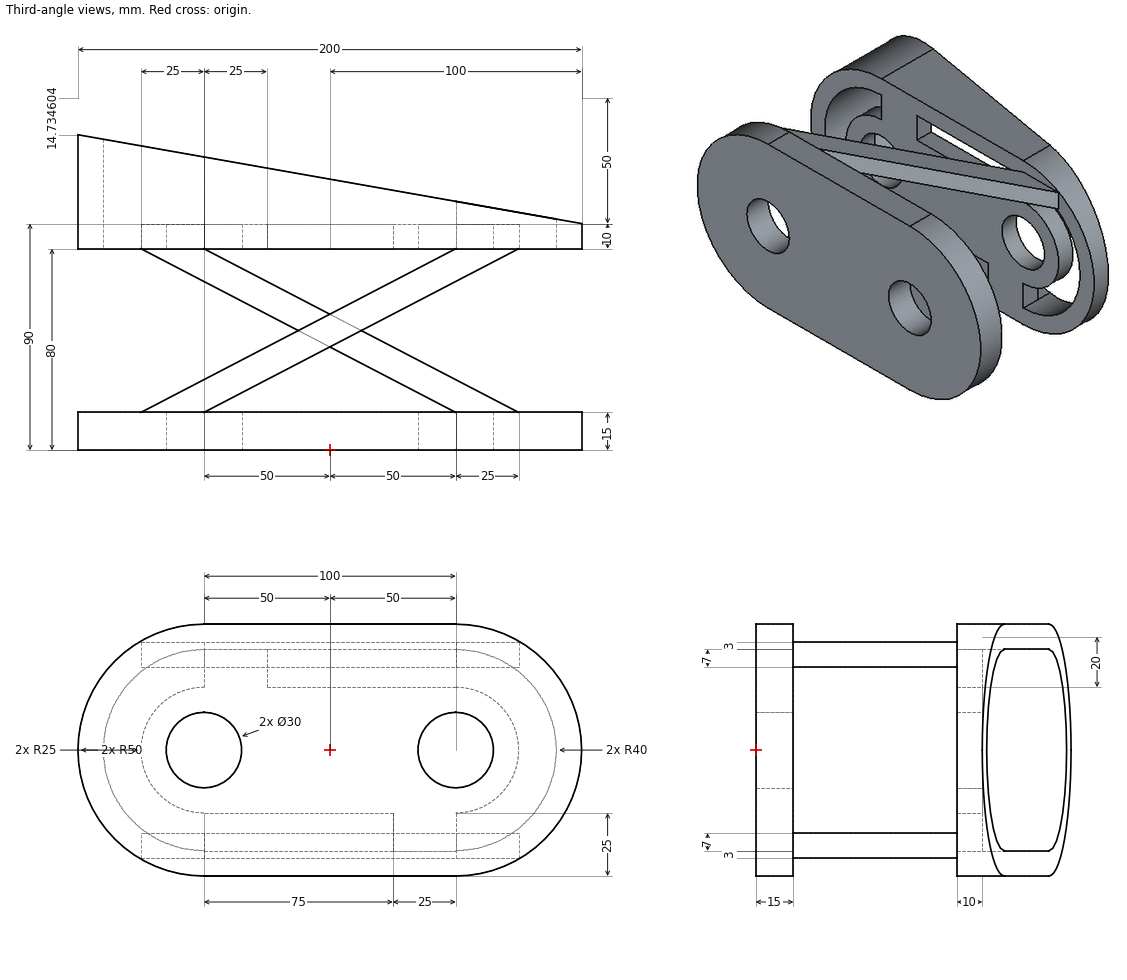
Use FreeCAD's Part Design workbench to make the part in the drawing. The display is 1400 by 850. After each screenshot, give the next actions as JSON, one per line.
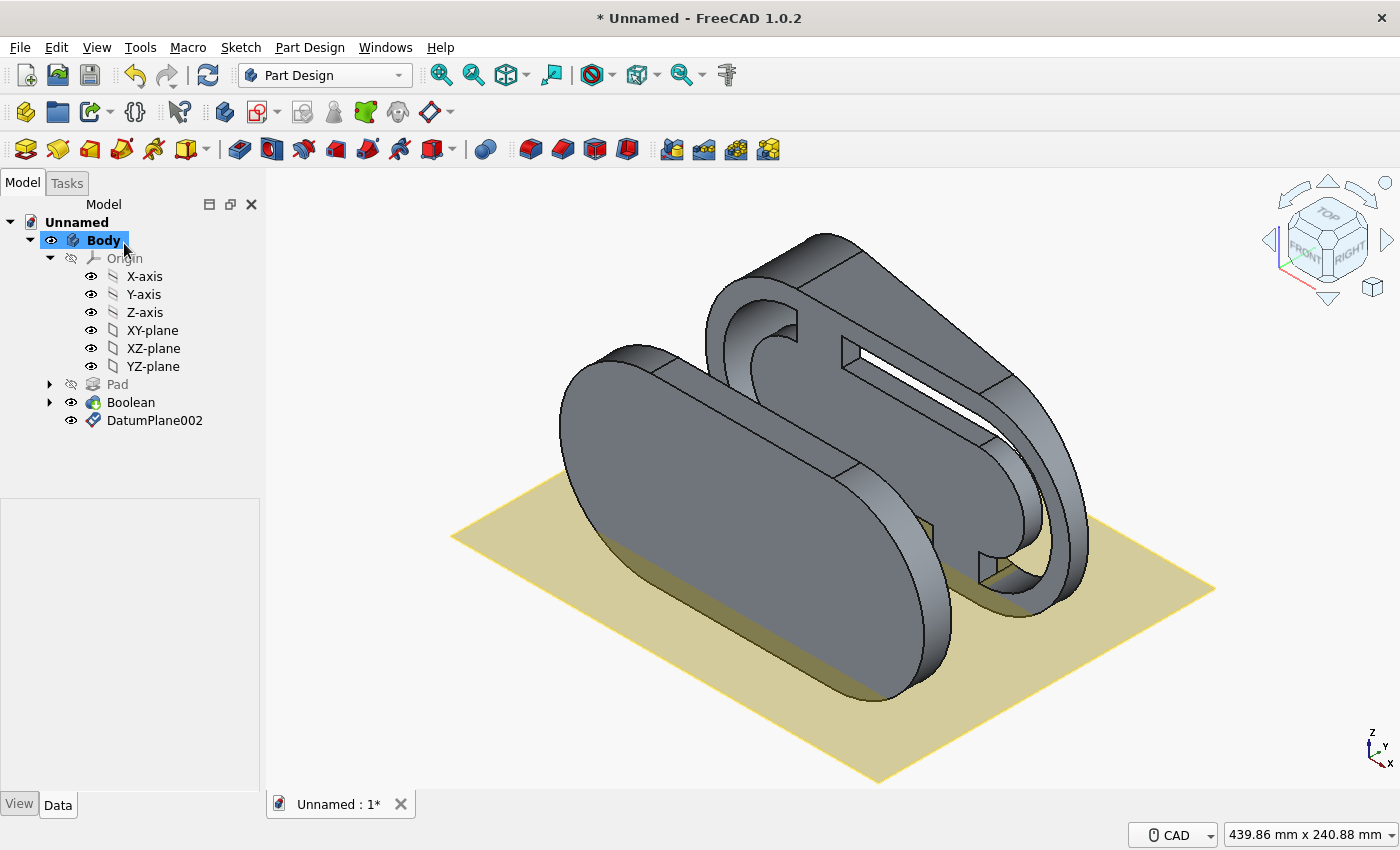
{"action": "left_click", "coordinate": [116, 420]}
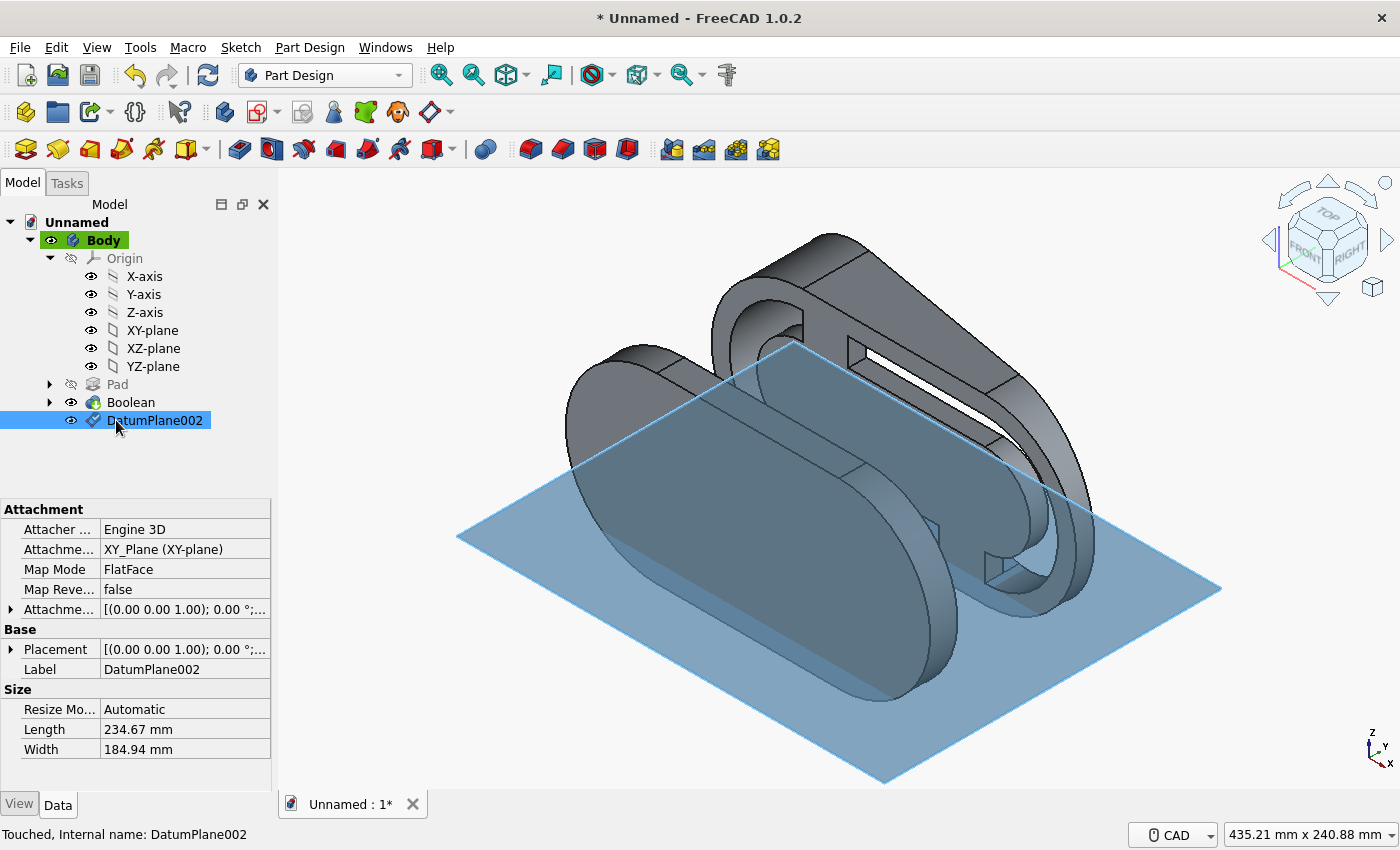
{"action": "left_click", "coordinate": [258, 112]}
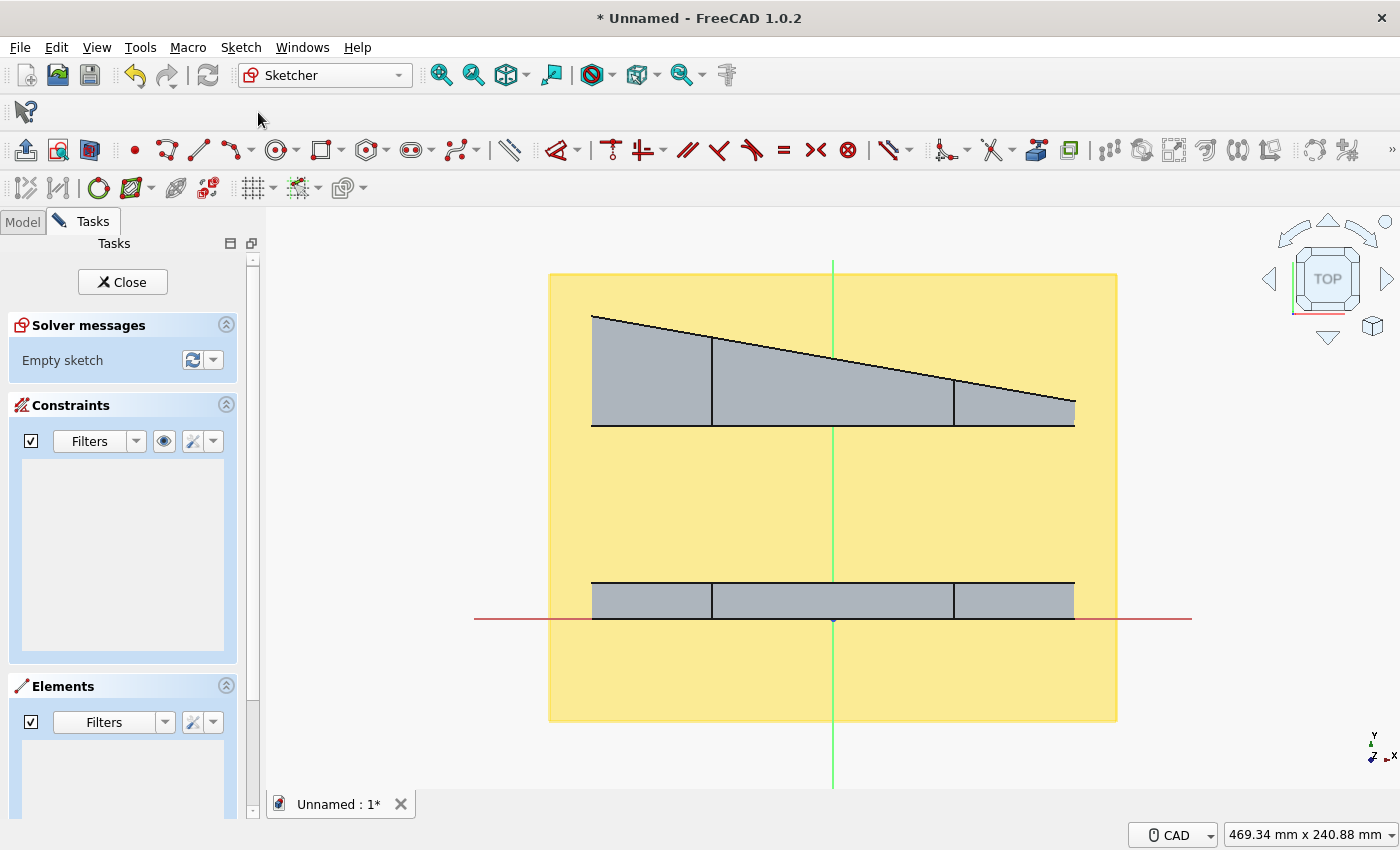
{"action": "left_click", "coordinate": [90, 150]}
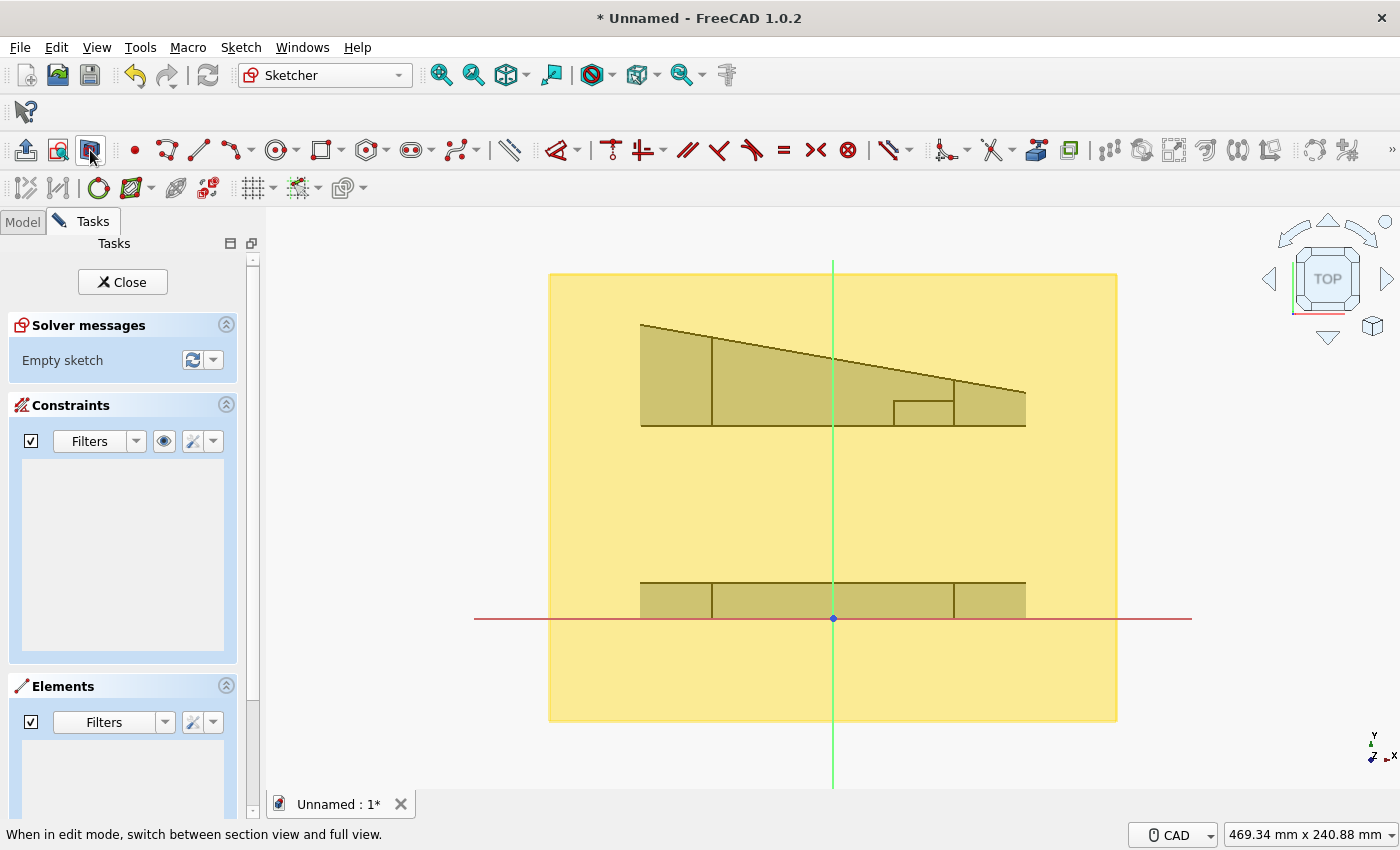
{"action": "scroll", "coordinate": [917, 552], "scroll_direction": "up", "scroll_amount": 3}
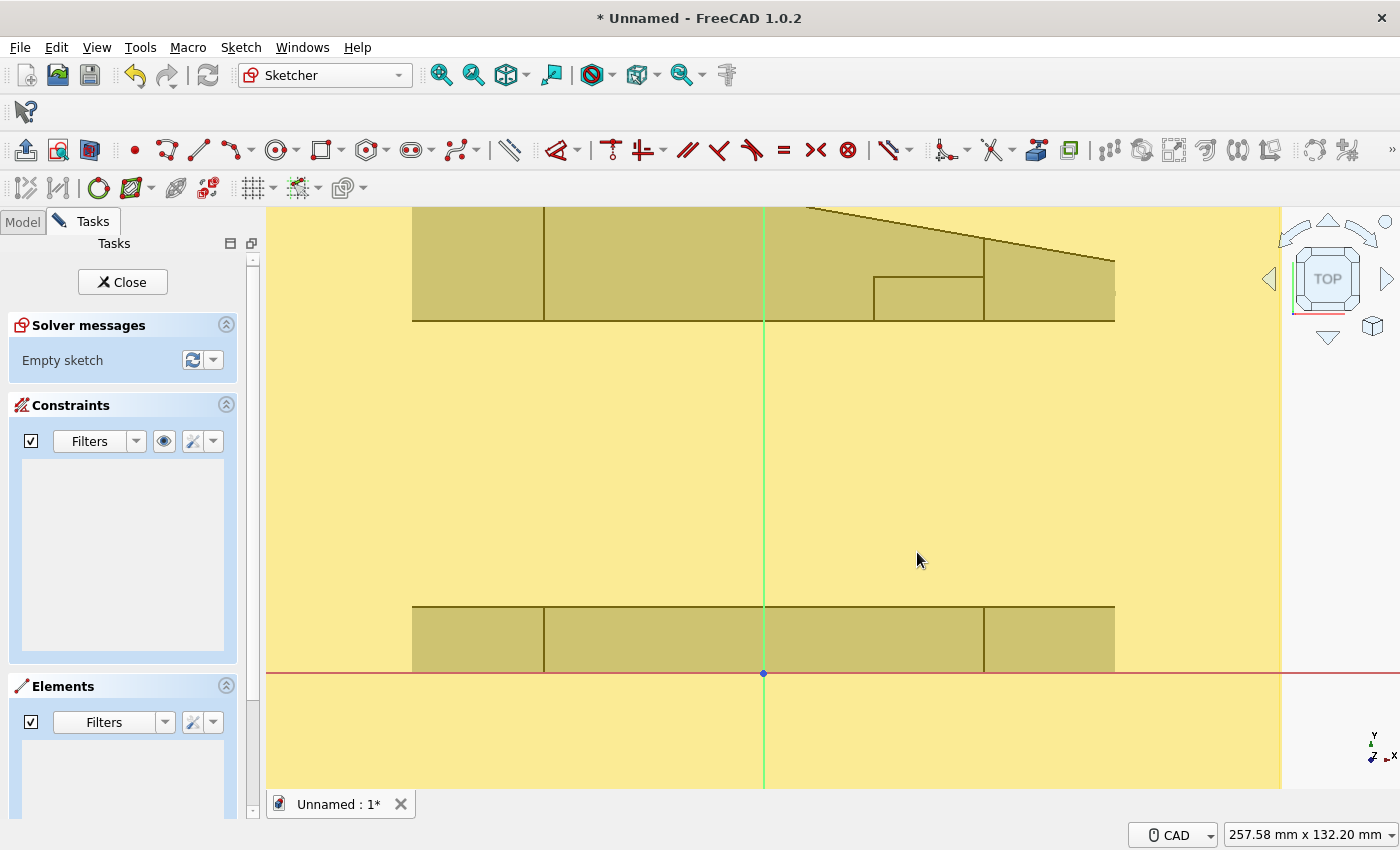
{"action": "left_click", "coordinate": [168, 150]}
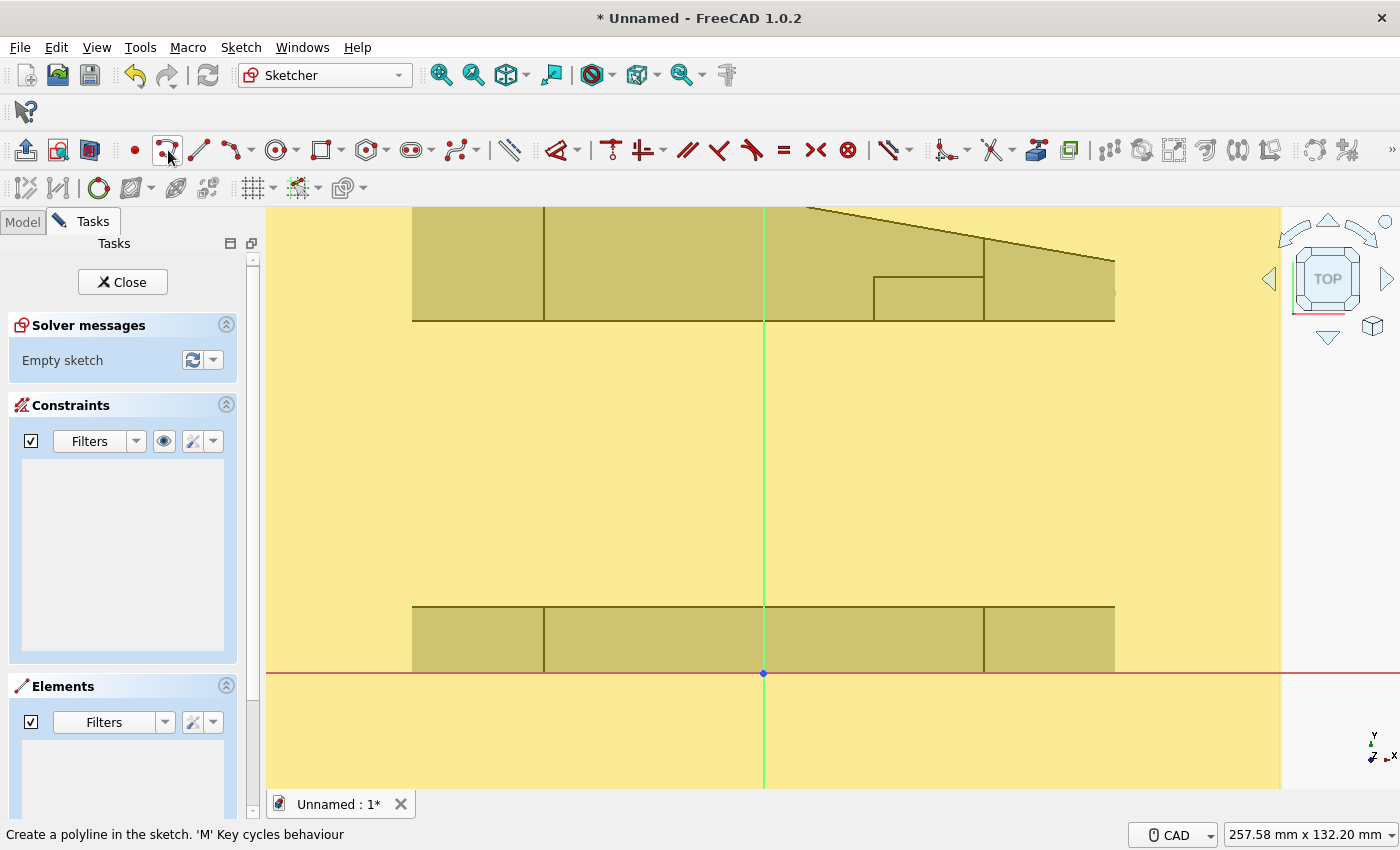
{"action": "left_click", "coordinate": [984, 607]}
{"action": "left_click", "coordinate": [1094, 607]}
{"action": "left_click", "coordinate": [544, 321]}
{"action": "left_click", "coordinate": [434, 321]}
{"action": "left_click", "coordinate": [984, 608]}
{"action": "key", "text": "Escape"}
{"action": "key", "text": "Escape"}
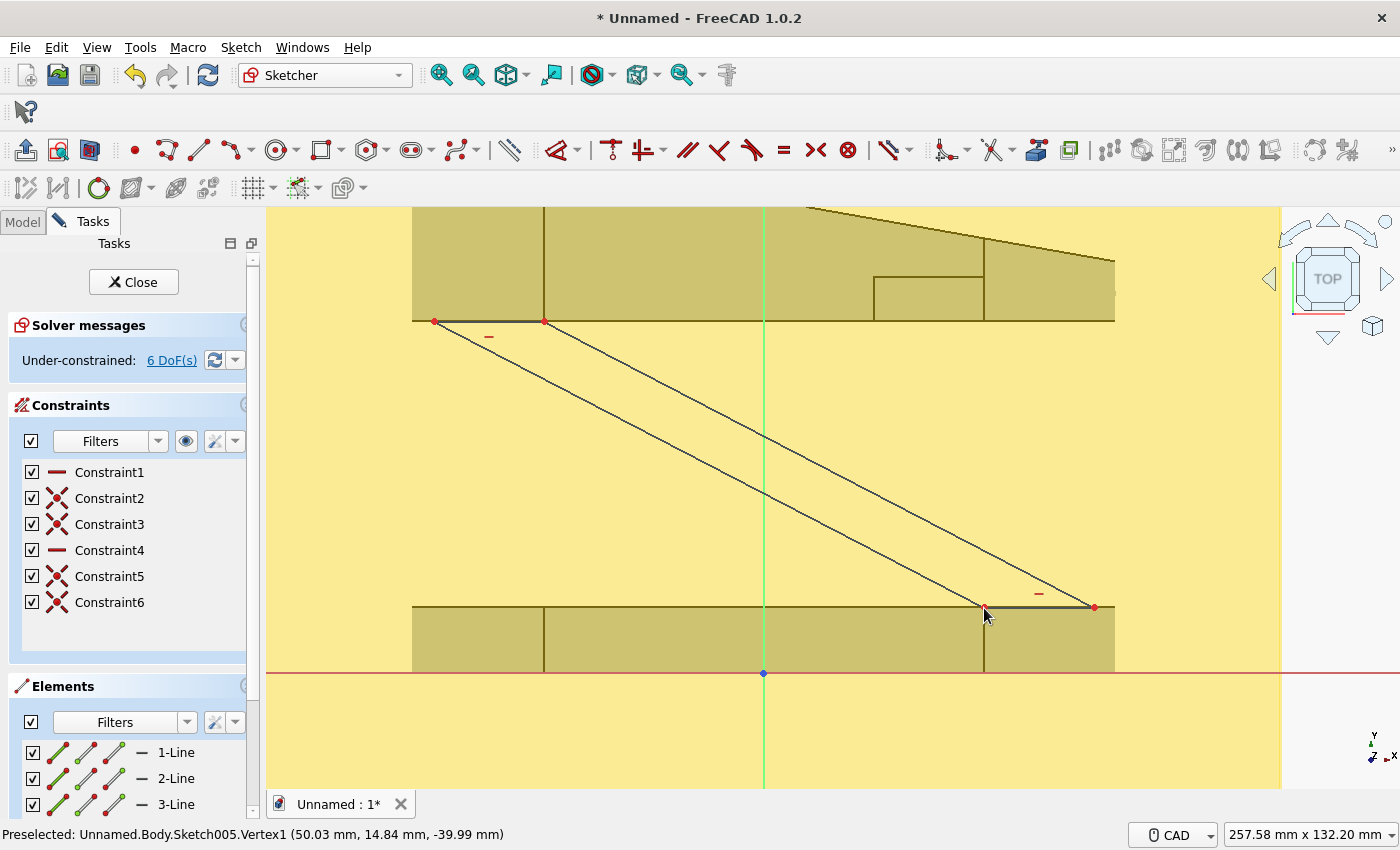
{"action": "left_click", "coordinate": [556, 150]}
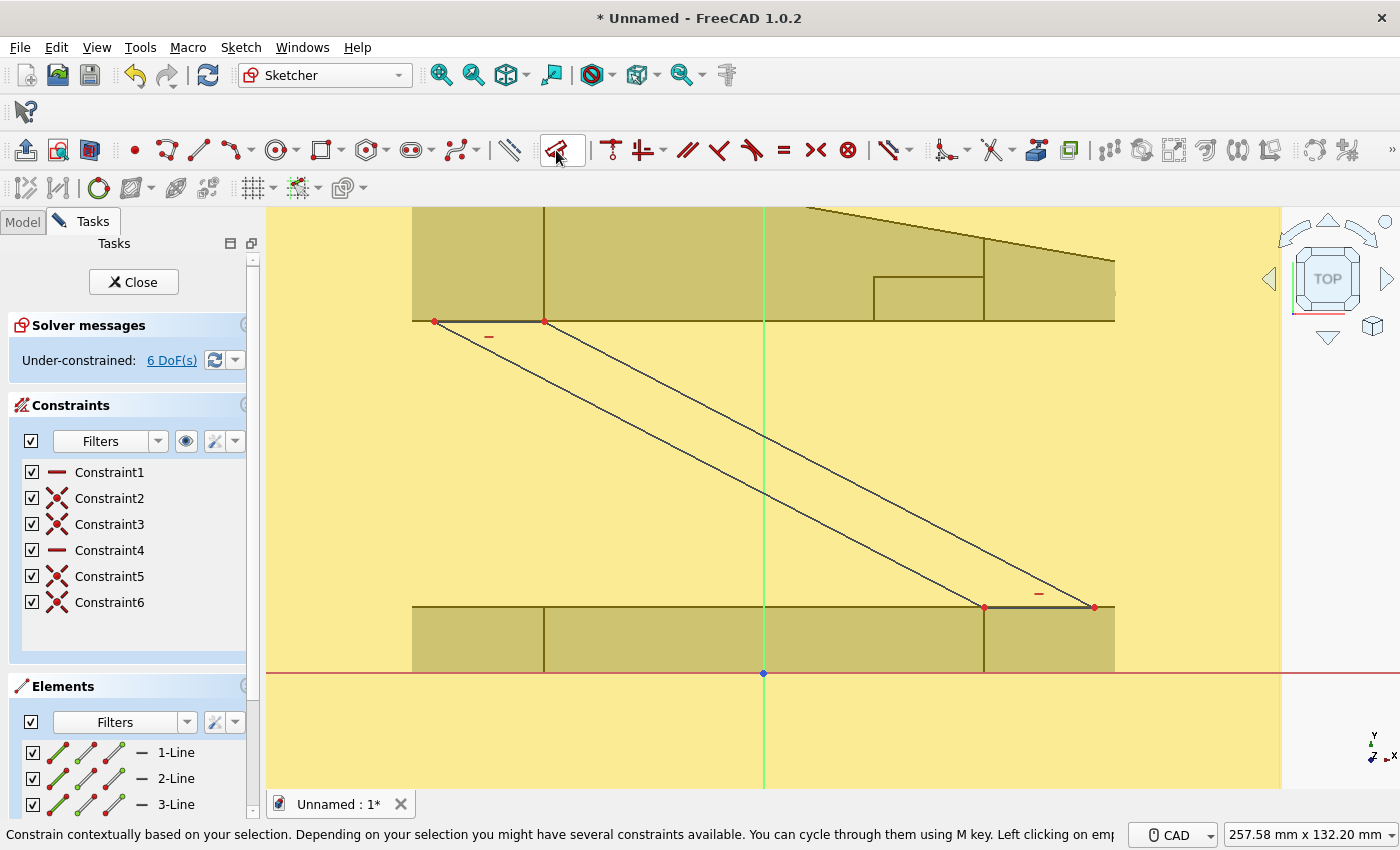
{"action": "left_click", "coordinate": [1017, 608]}
{"action": "left_click", "coordinate": [1039, 642]}